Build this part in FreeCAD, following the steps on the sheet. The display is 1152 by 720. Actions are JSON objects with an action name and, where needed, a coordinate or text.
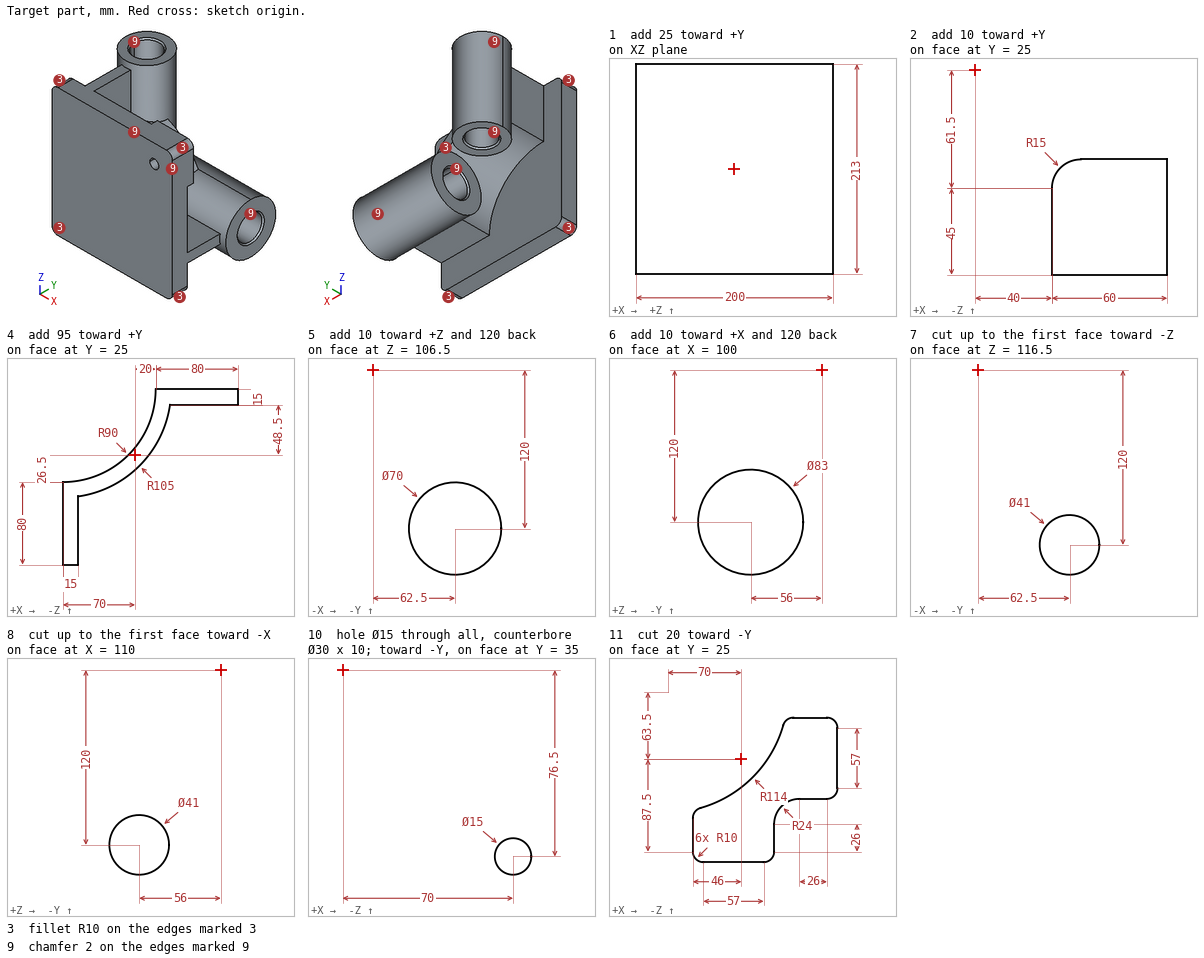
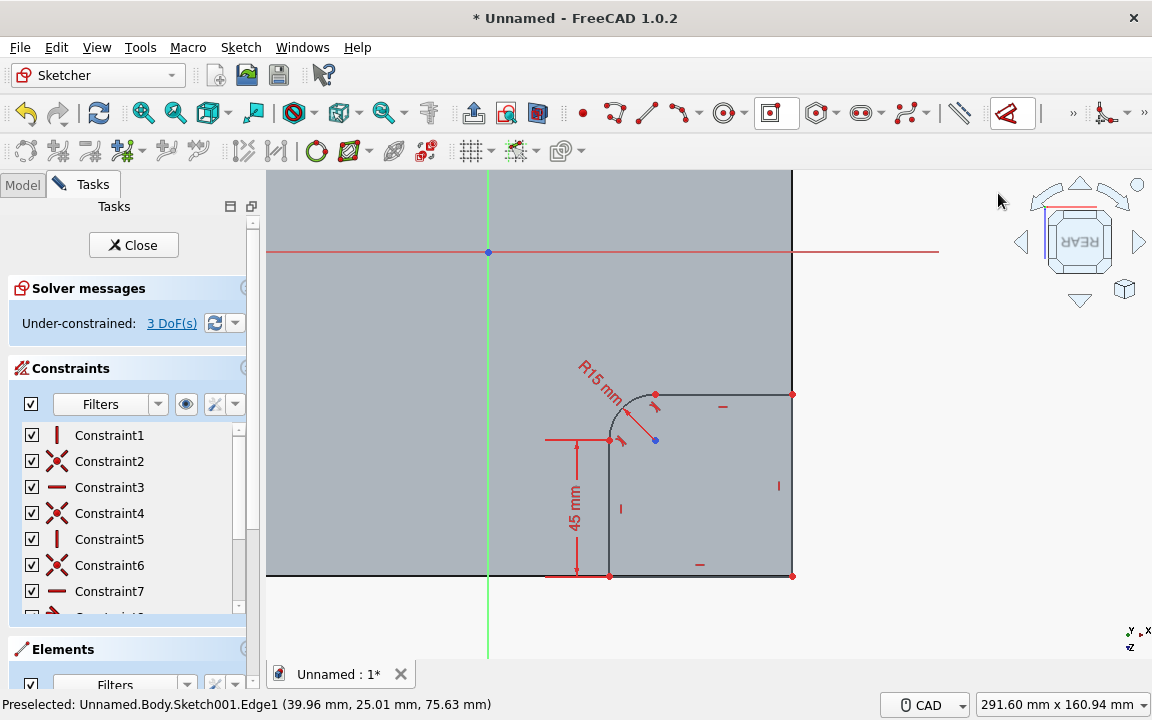
{"action": "left_click", "coordinate": [664, 577]}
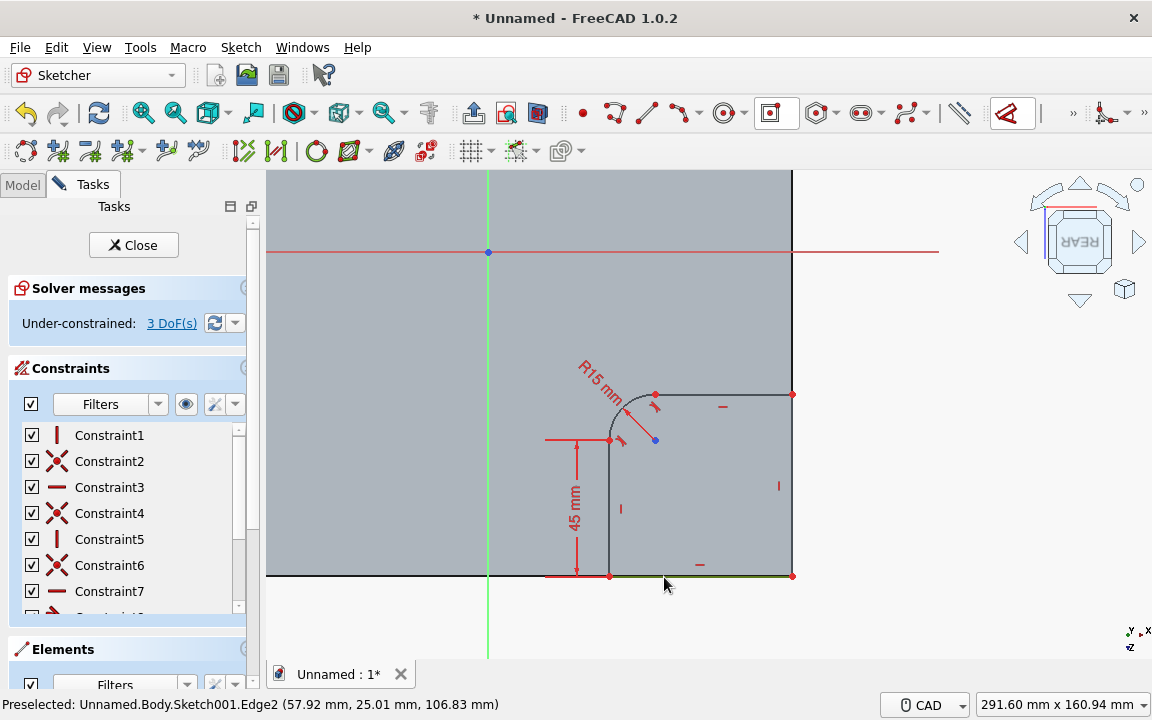
{"action": "left_click", "coordinate": [1030, 114]}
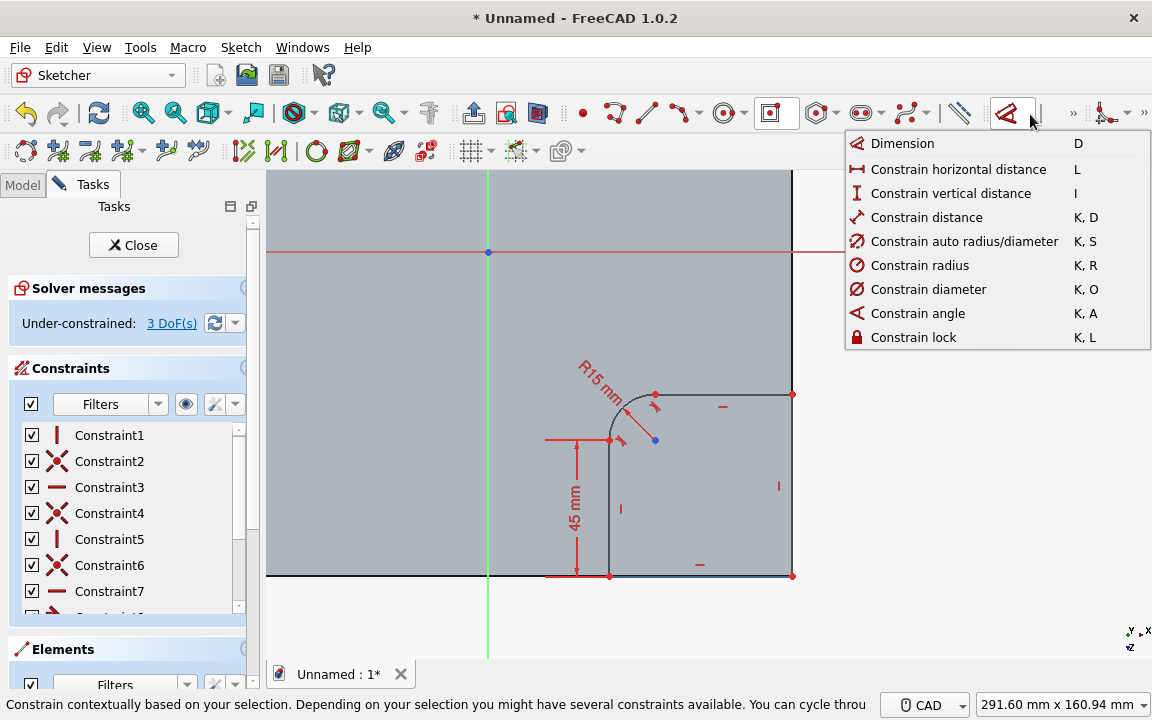
{"action": "left_click", "coordinate": [998, 169]}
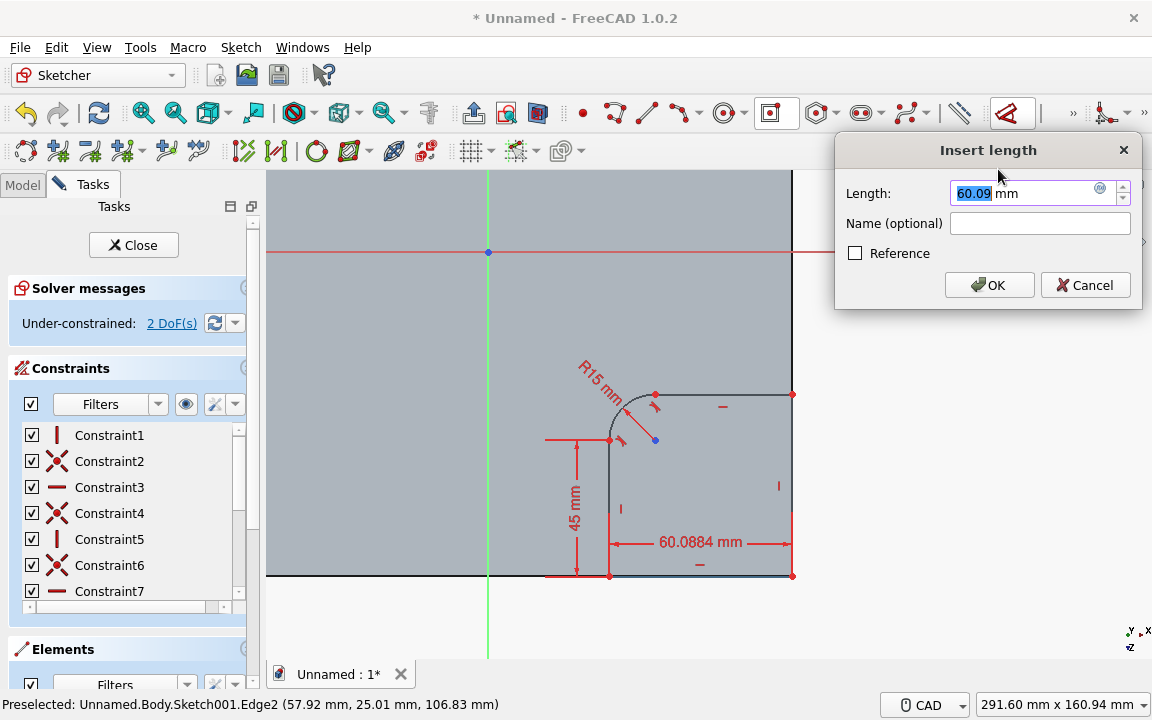
{"action": "type", "text": "60"}
{"action": "key", "text": "Return"}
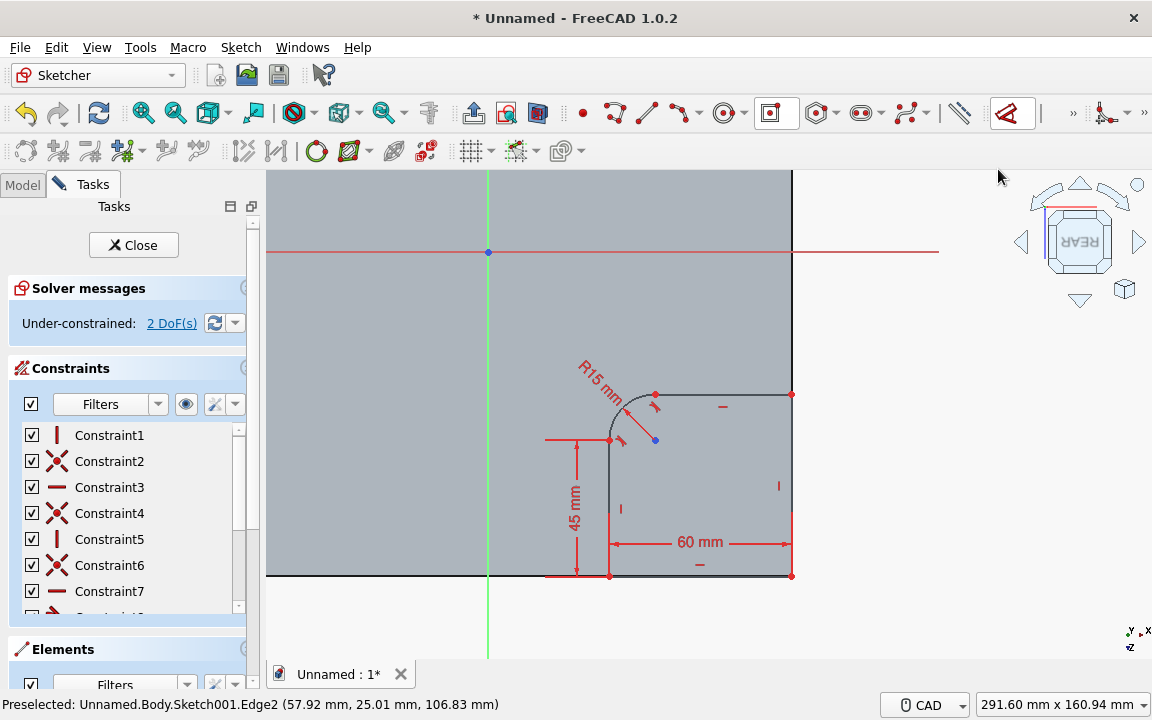
{"action": "left_click", "coordinate": [609, 440]}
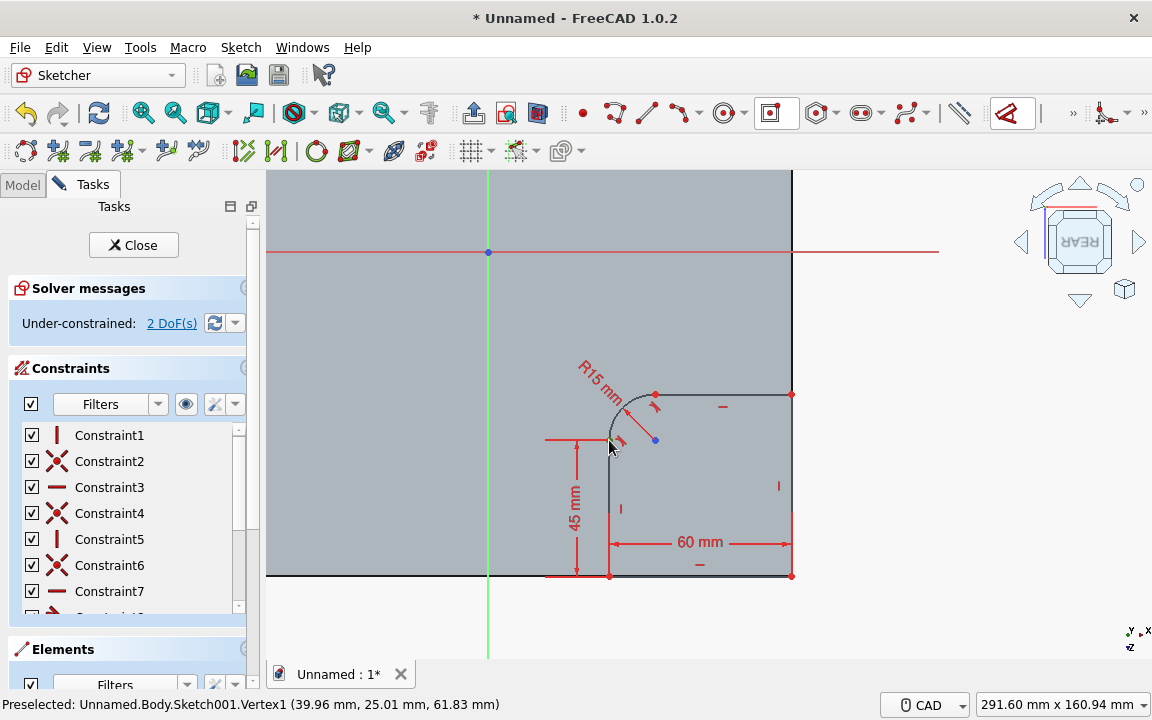
{"action": "left_click", "coordinate": [1030, 114]}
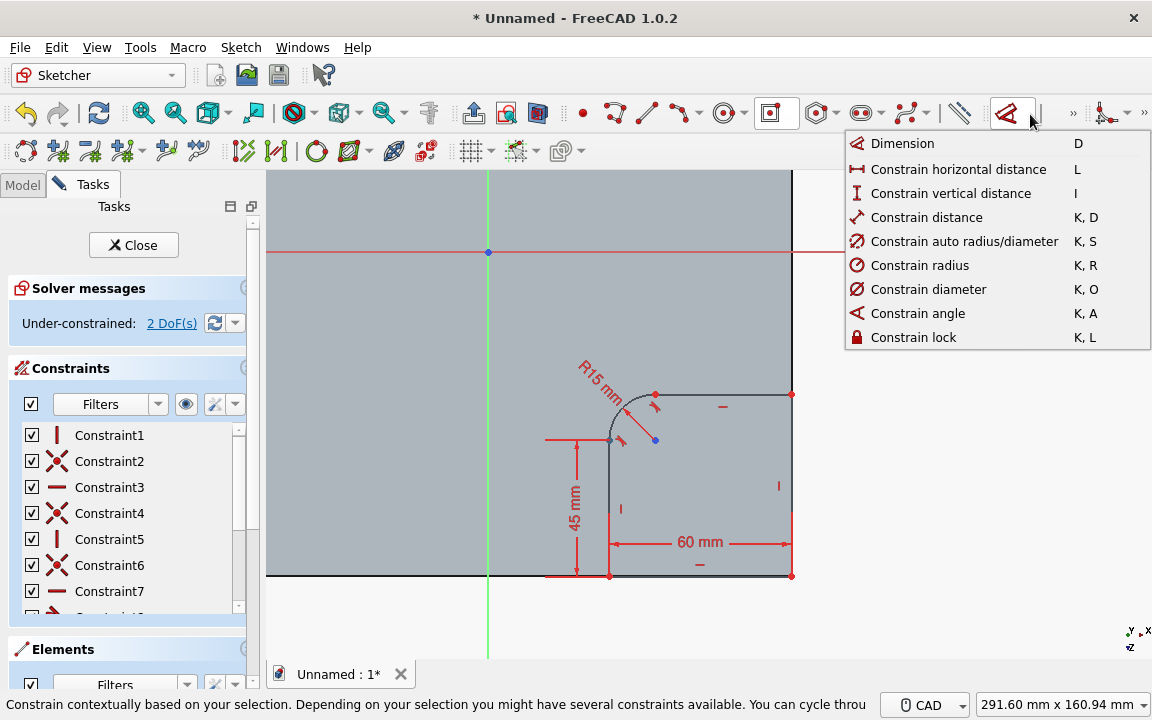
{"action": "left_click", "coordinate": [998, 169]}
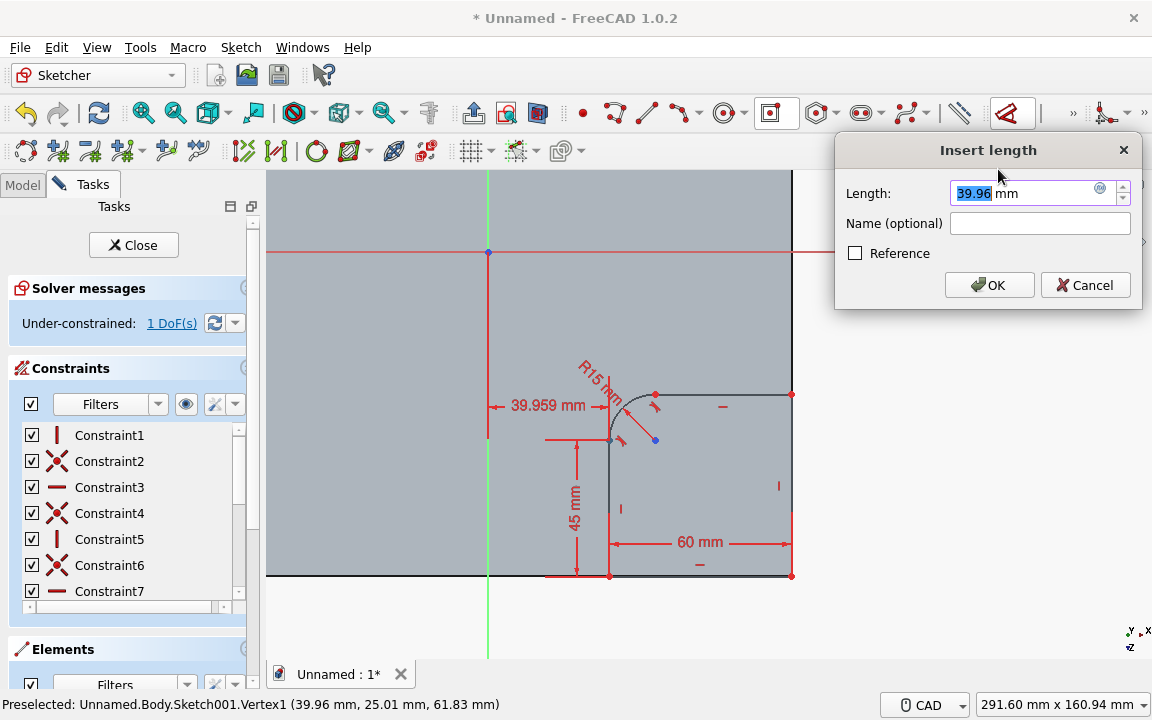
{"action": "type", "text": "40"}
{"action": "key", "text": "Return"}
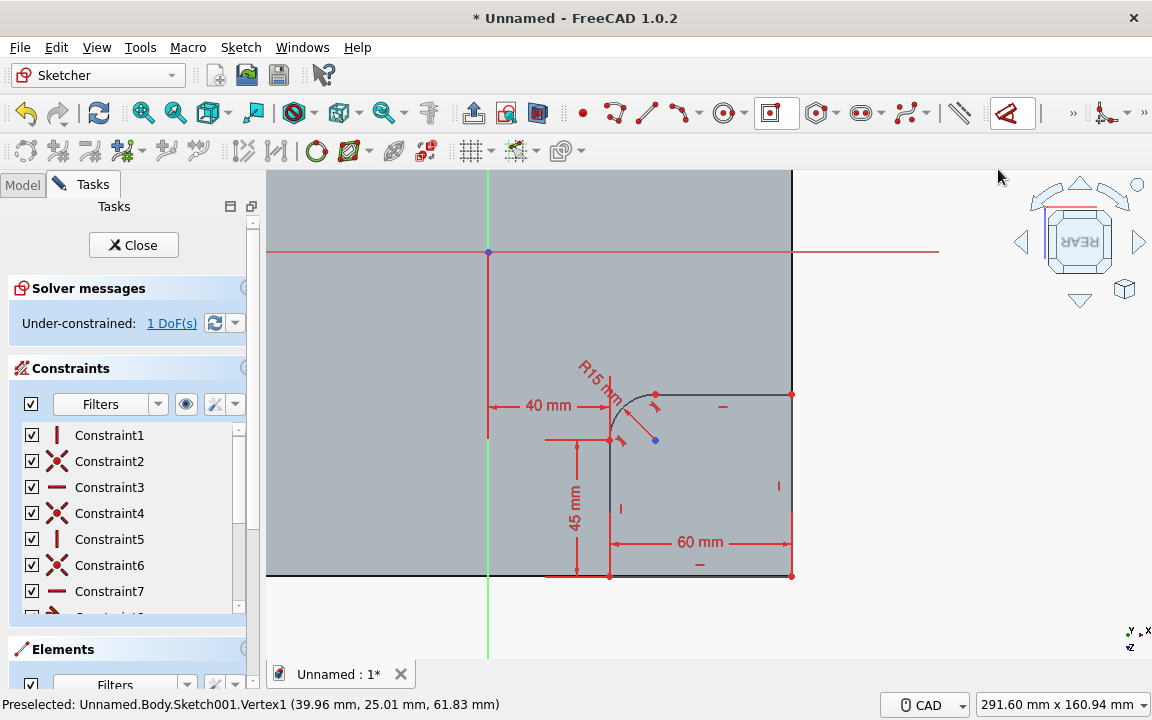
{"action": "left_click", "coordinate": [610, 440]}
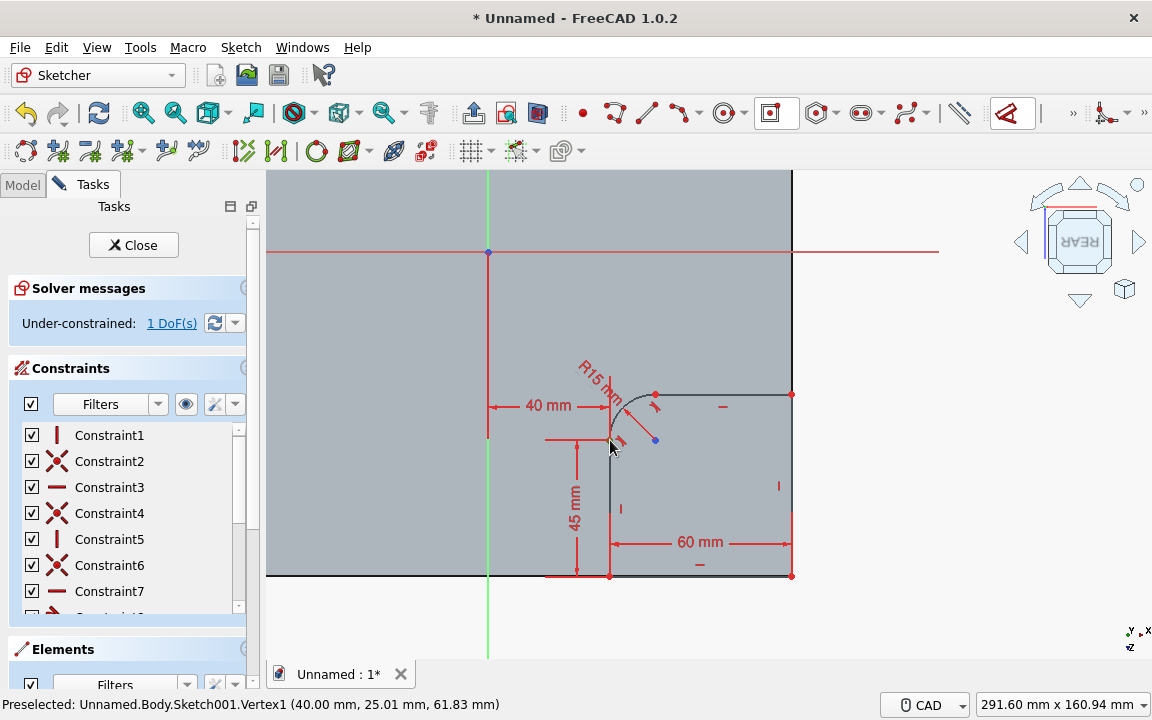
{"action": "key", "text": "i"}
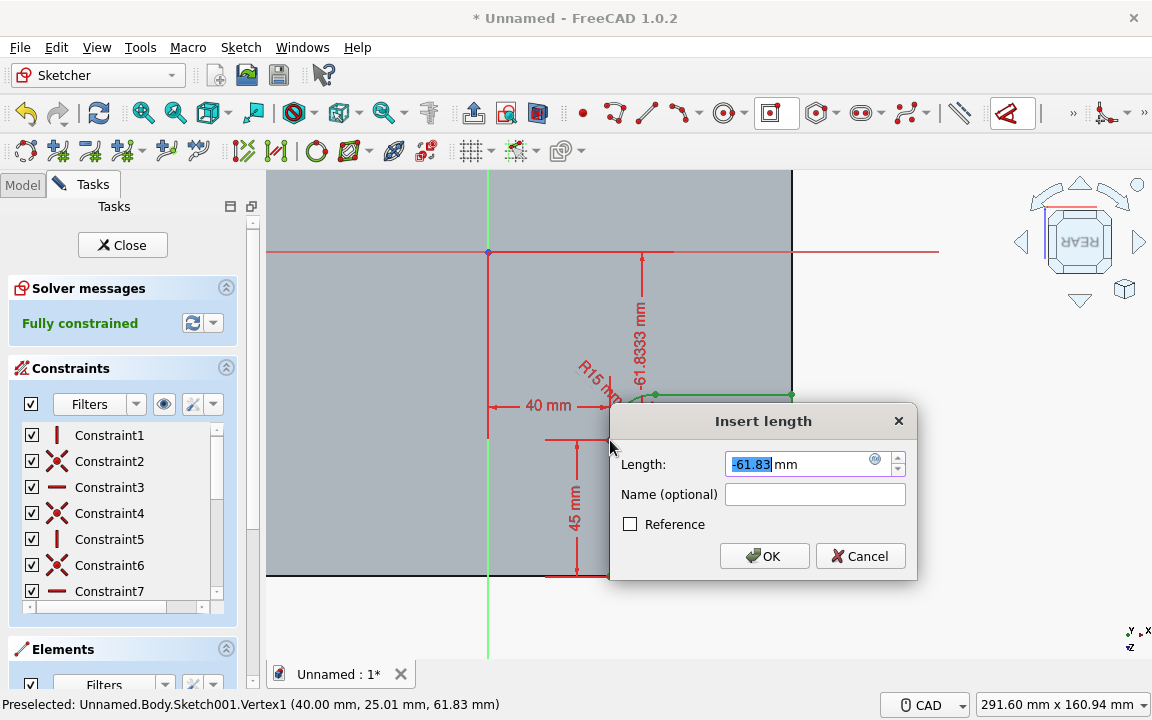
{"action": "type", "text": "-61.5"}
{"action": "key", "text": "Return"}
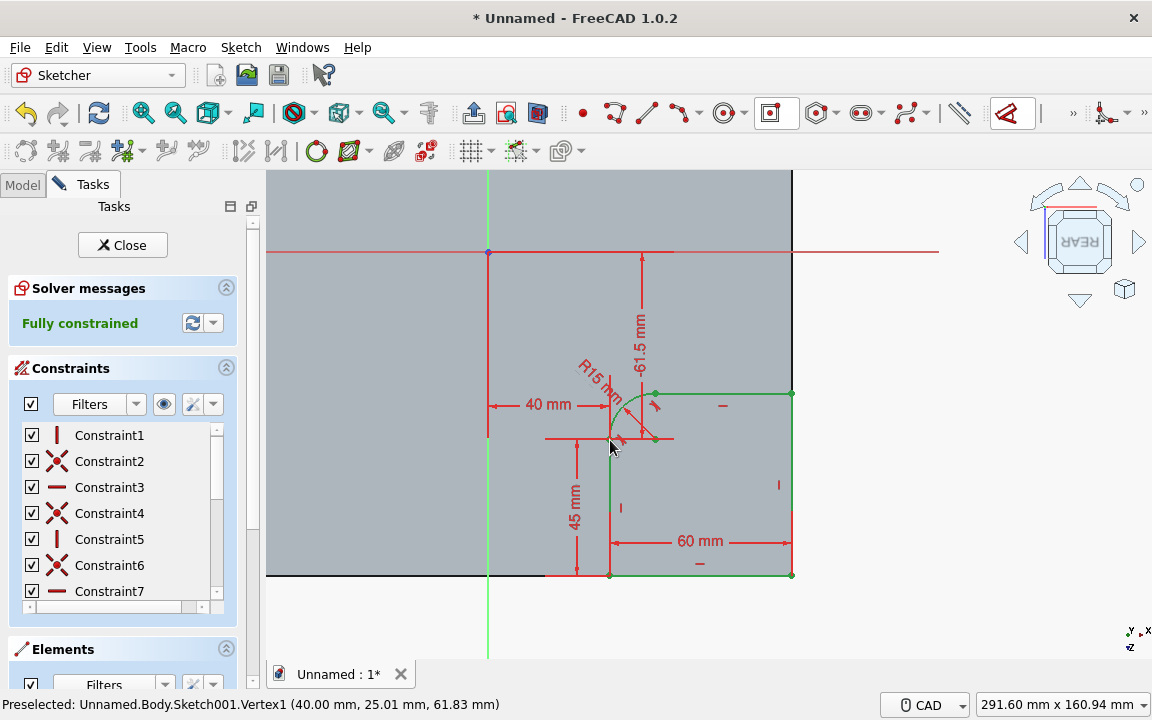
{"action": "left_click", "coordinate": [123, 245]}